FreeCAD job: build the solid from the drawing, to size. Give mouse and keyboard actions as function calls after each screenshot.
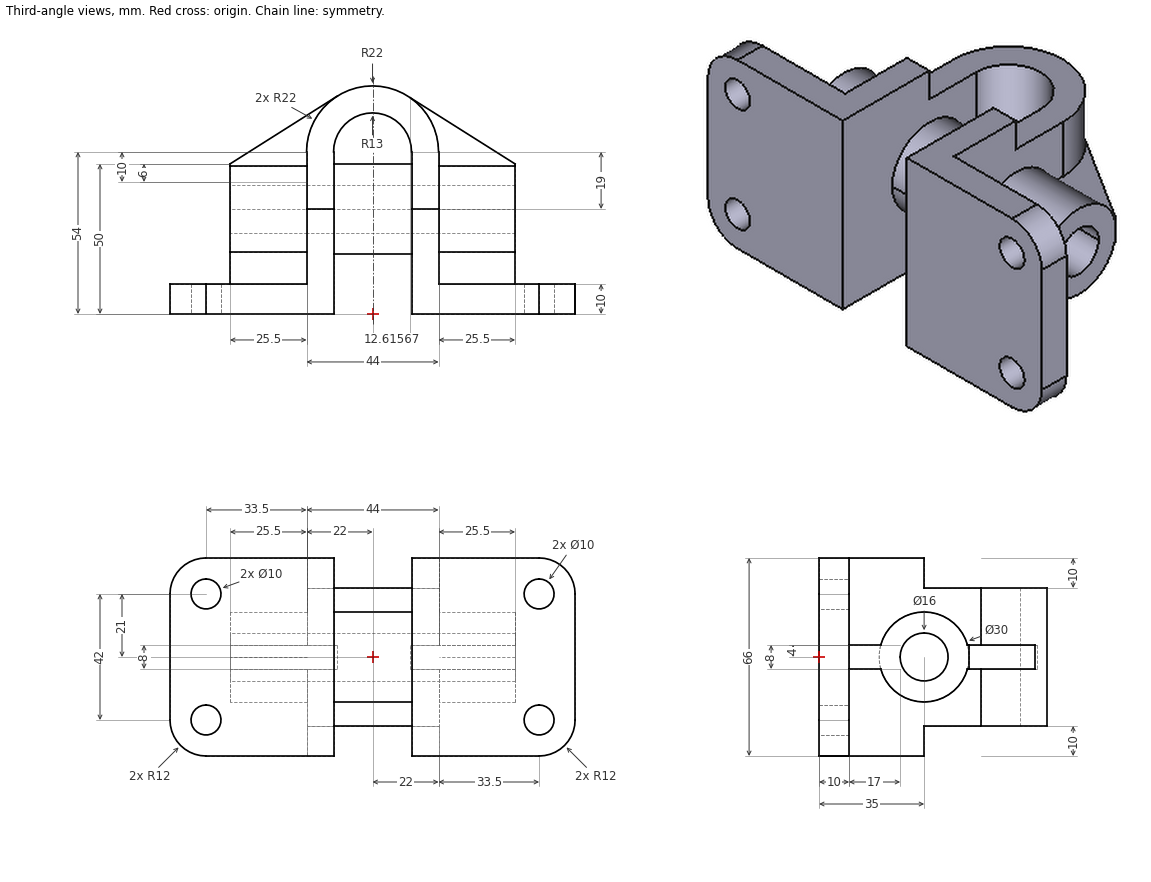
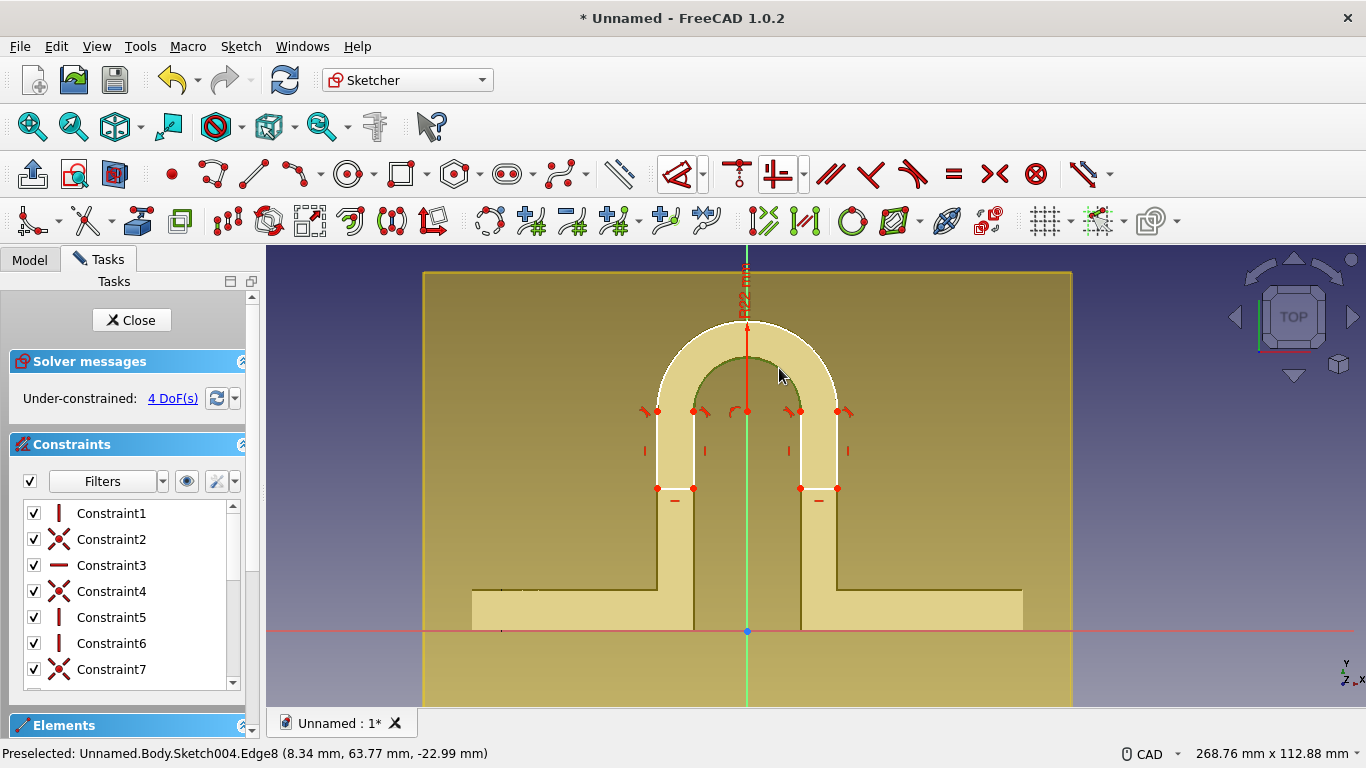
click(702, 174)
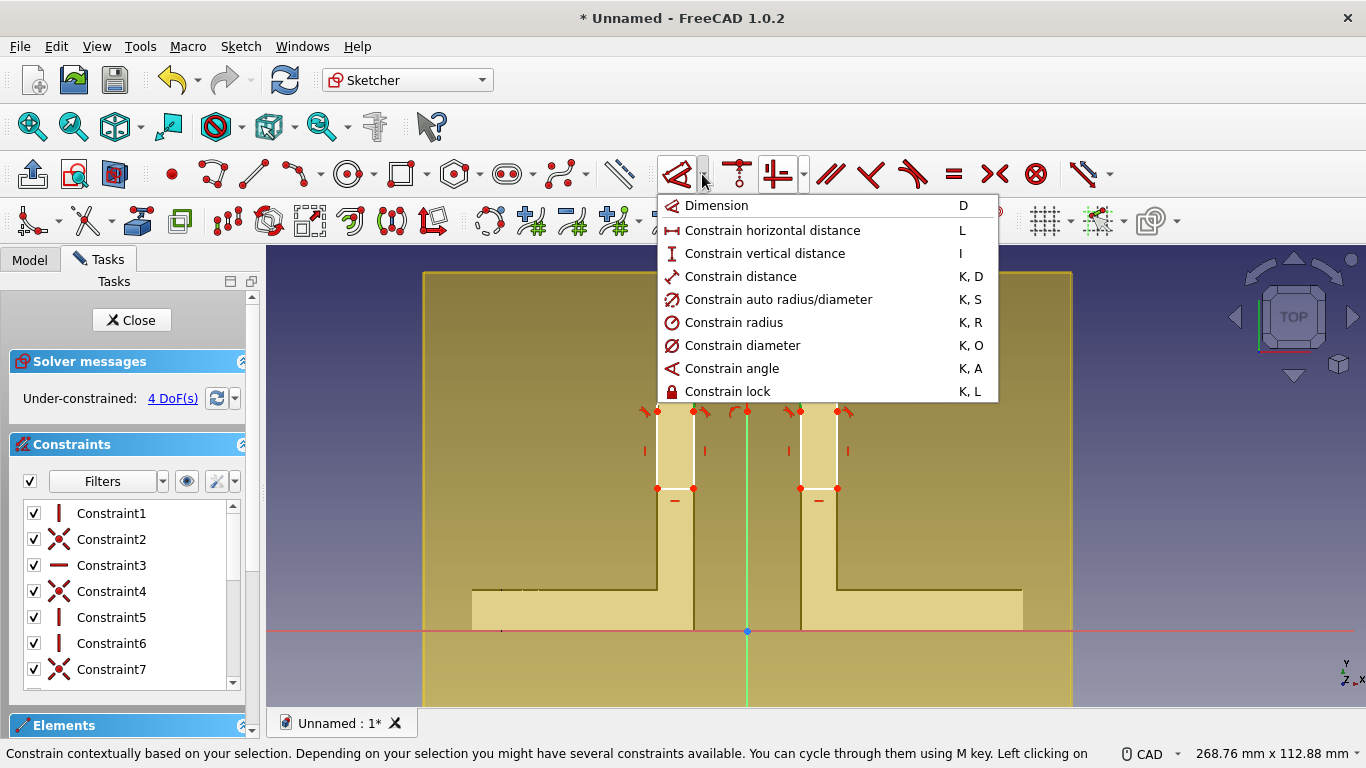
click(828, 322)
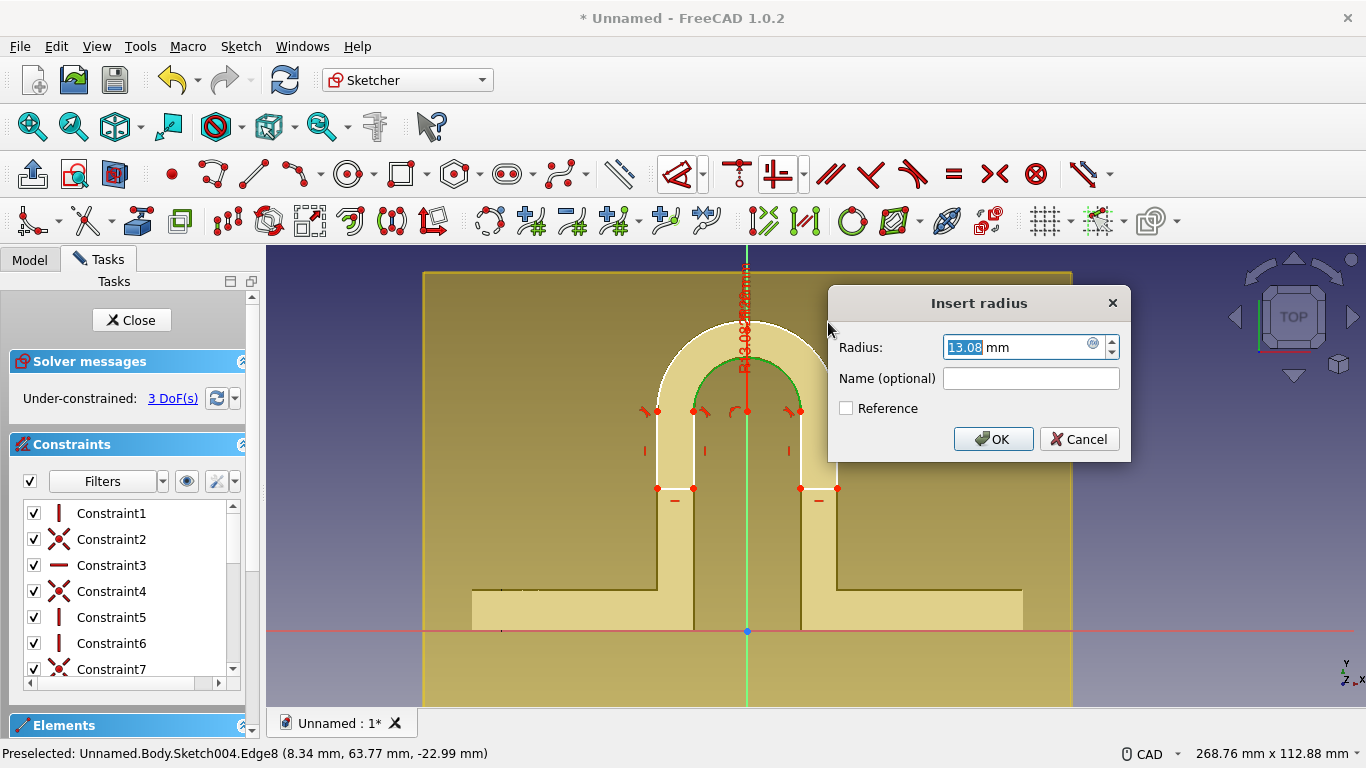
text(13)
key(Return)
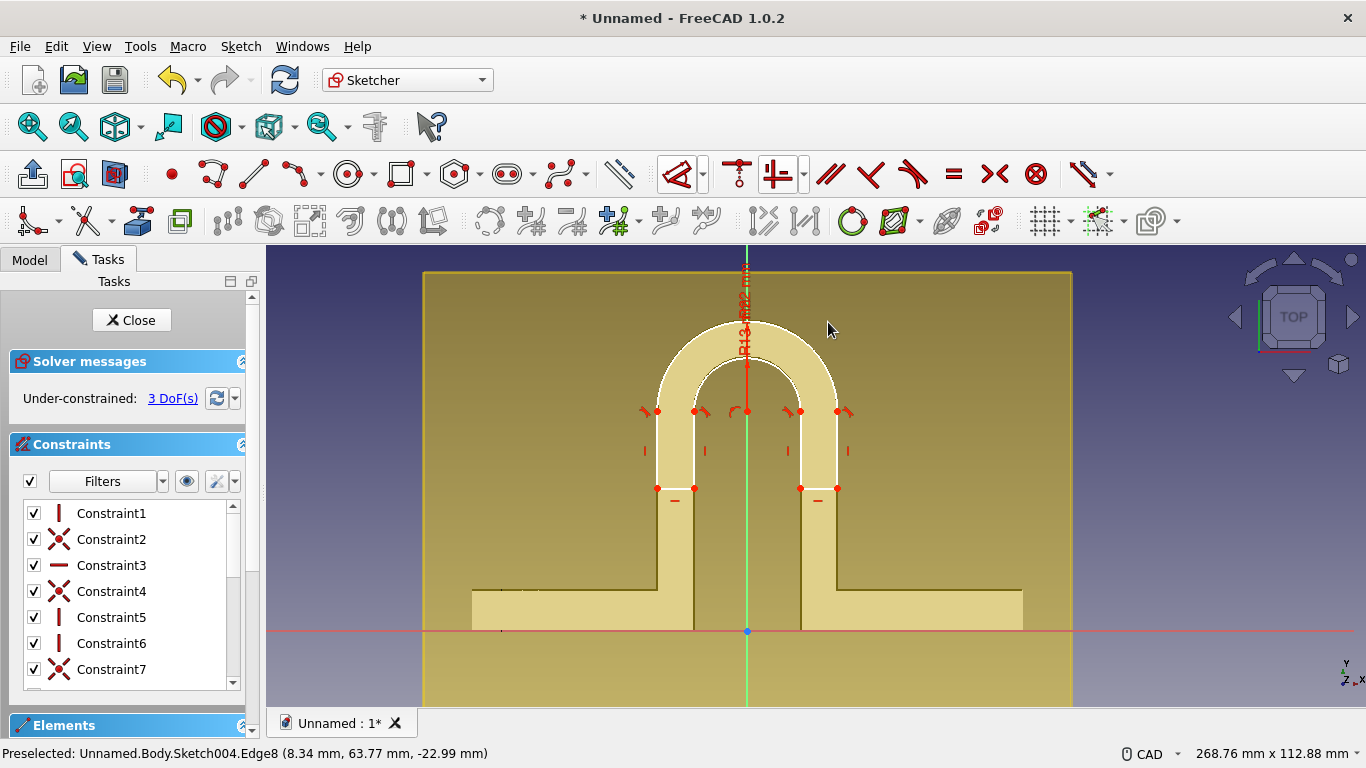
click(694, 435)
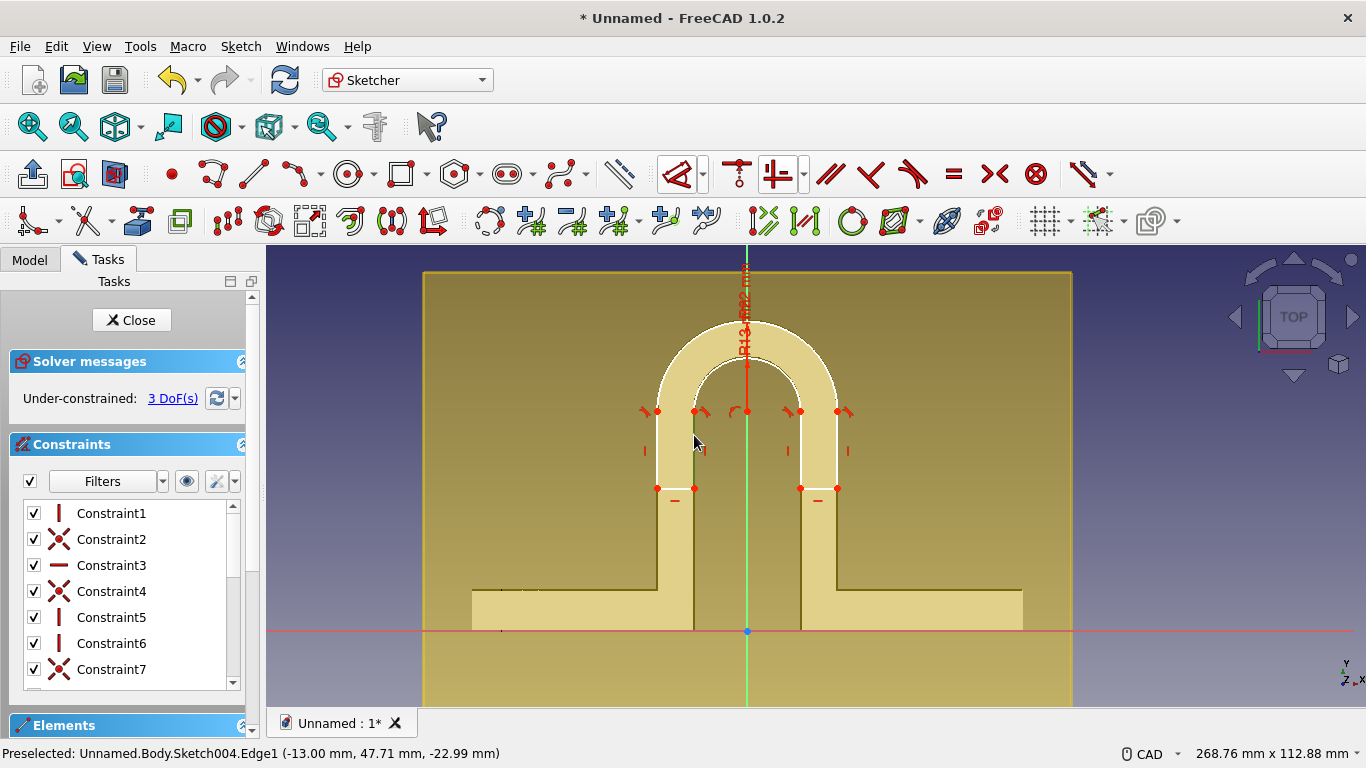
click(702, 174)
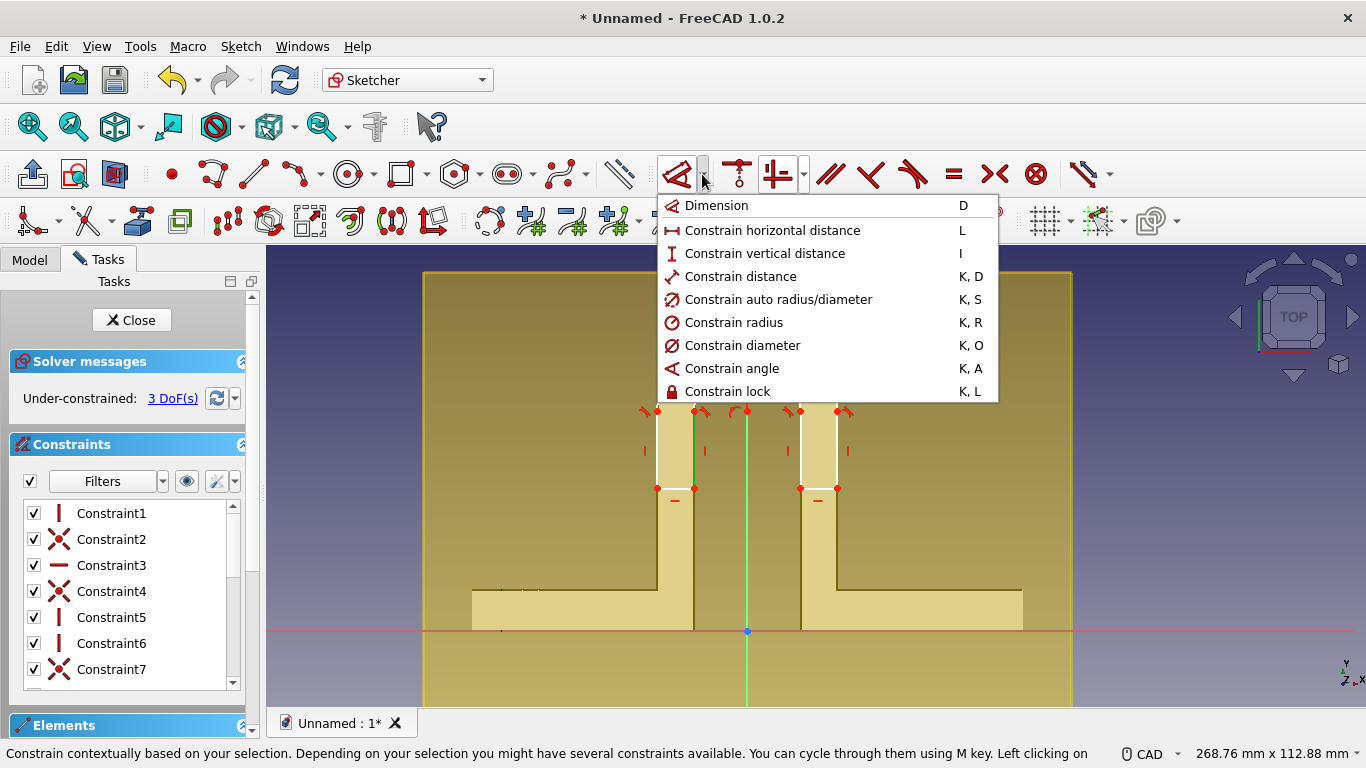
click(828, 254)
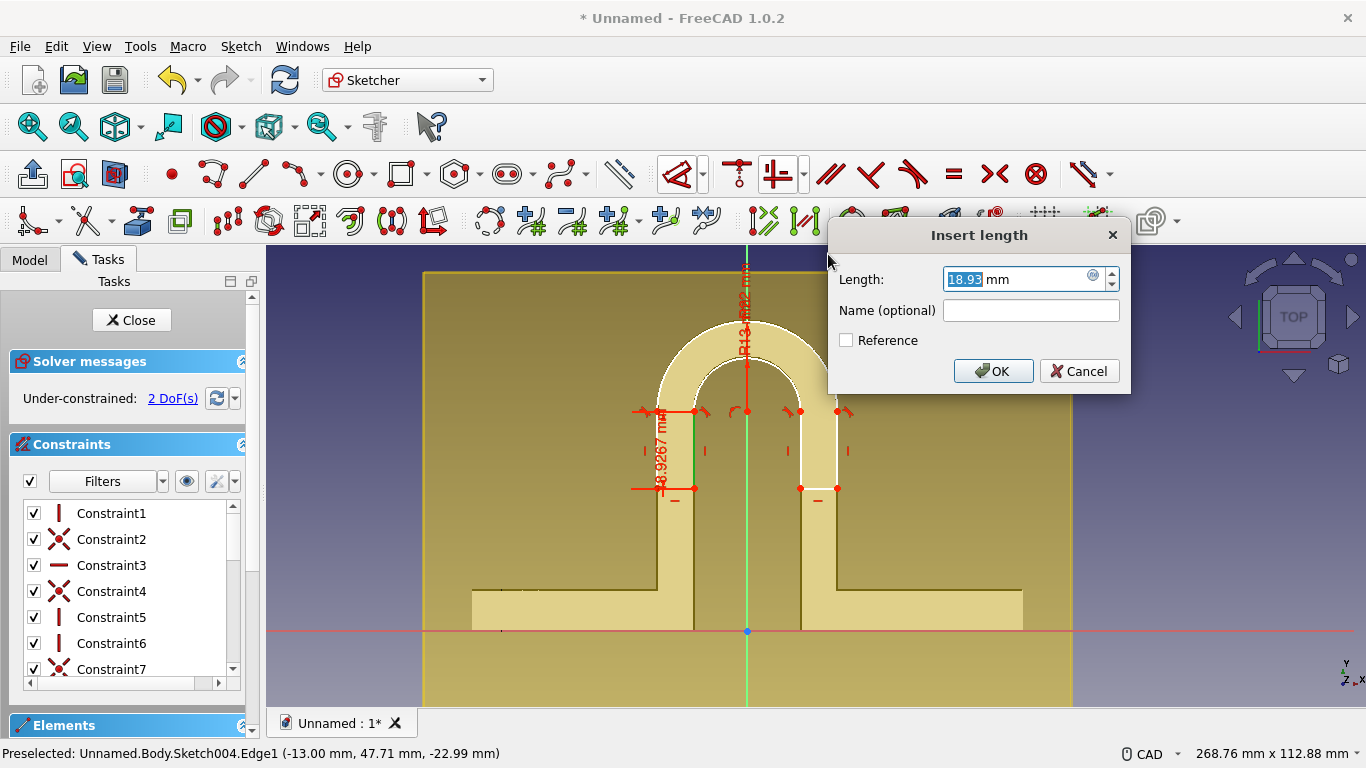
text(19)
key(Return)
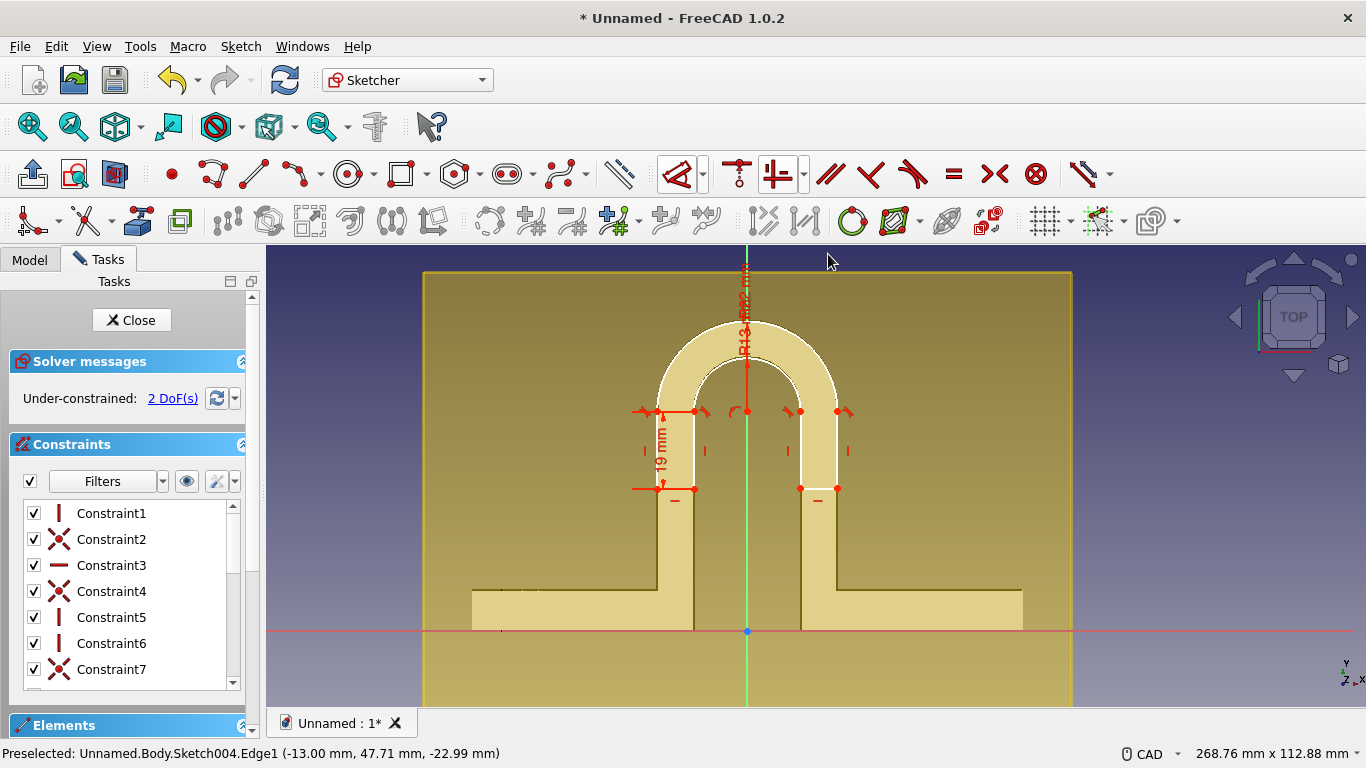
click(837, 435)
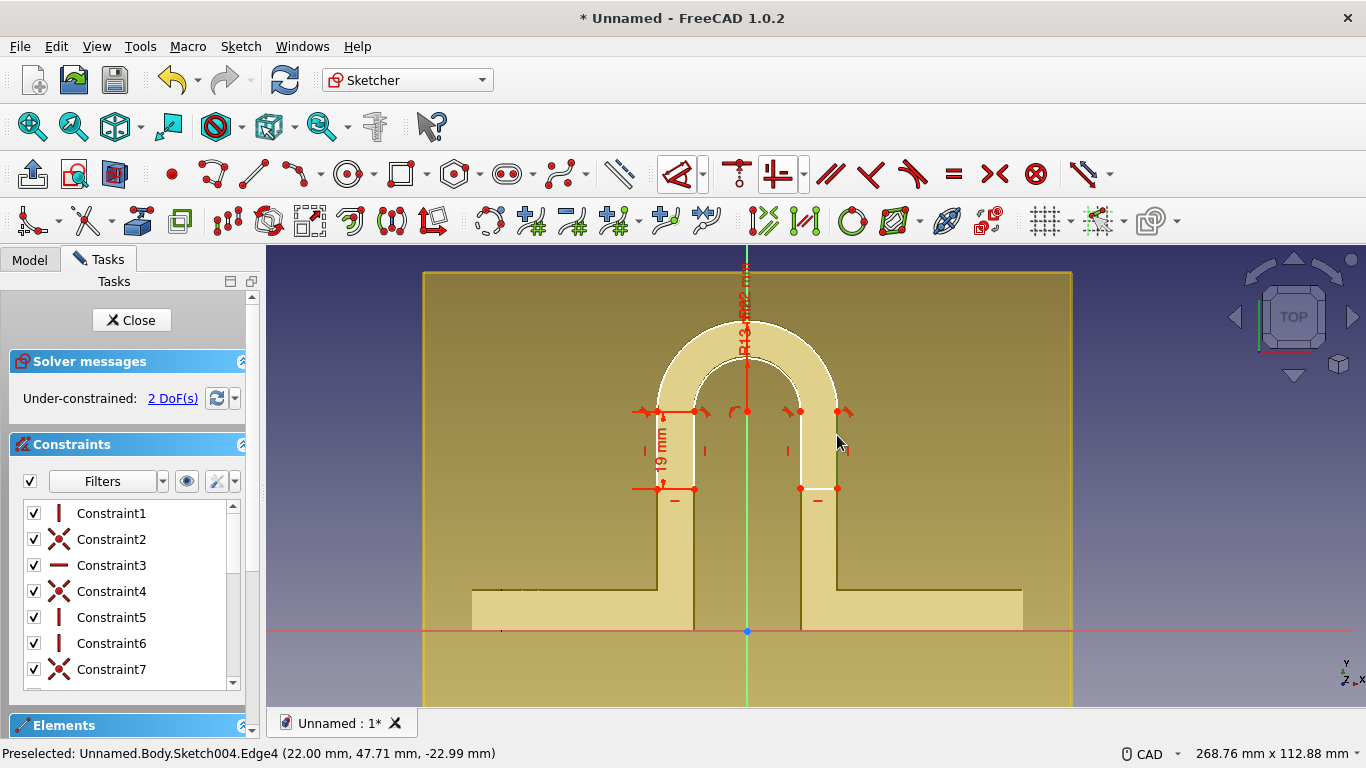
click(702, 174)